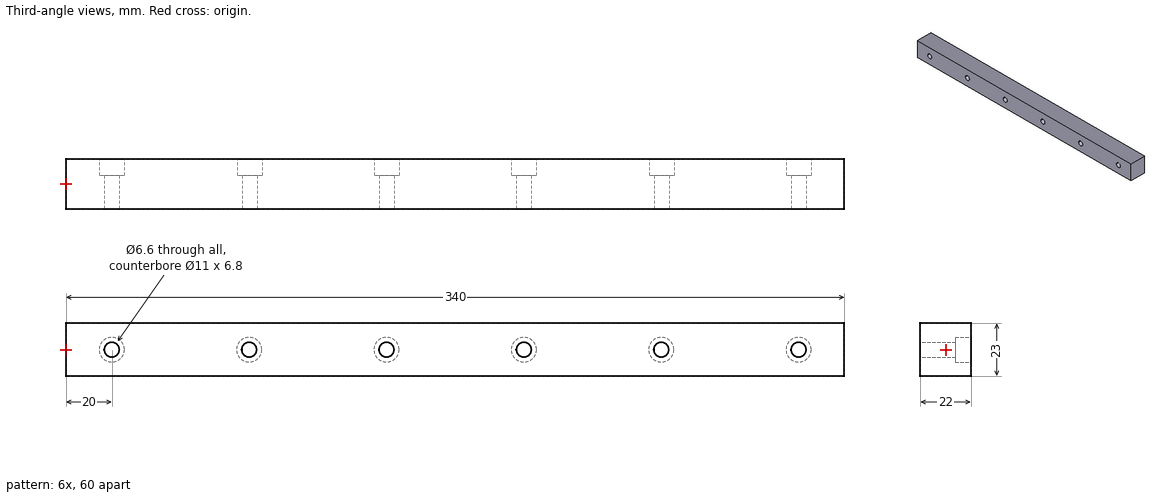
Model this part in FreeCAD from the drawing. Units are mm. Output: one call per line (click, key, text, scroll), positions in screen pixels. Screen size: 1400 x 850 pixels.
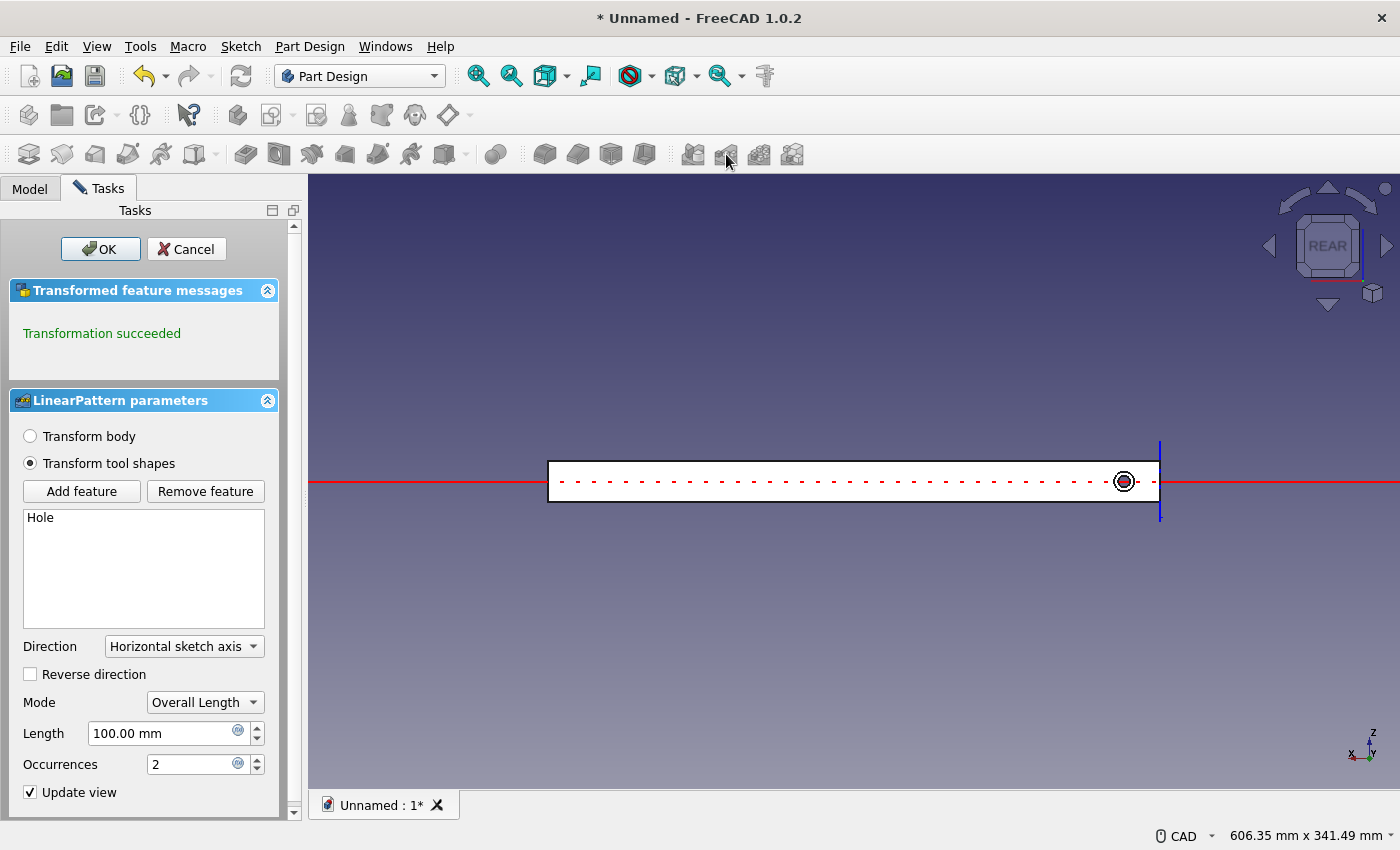
click(185, 646)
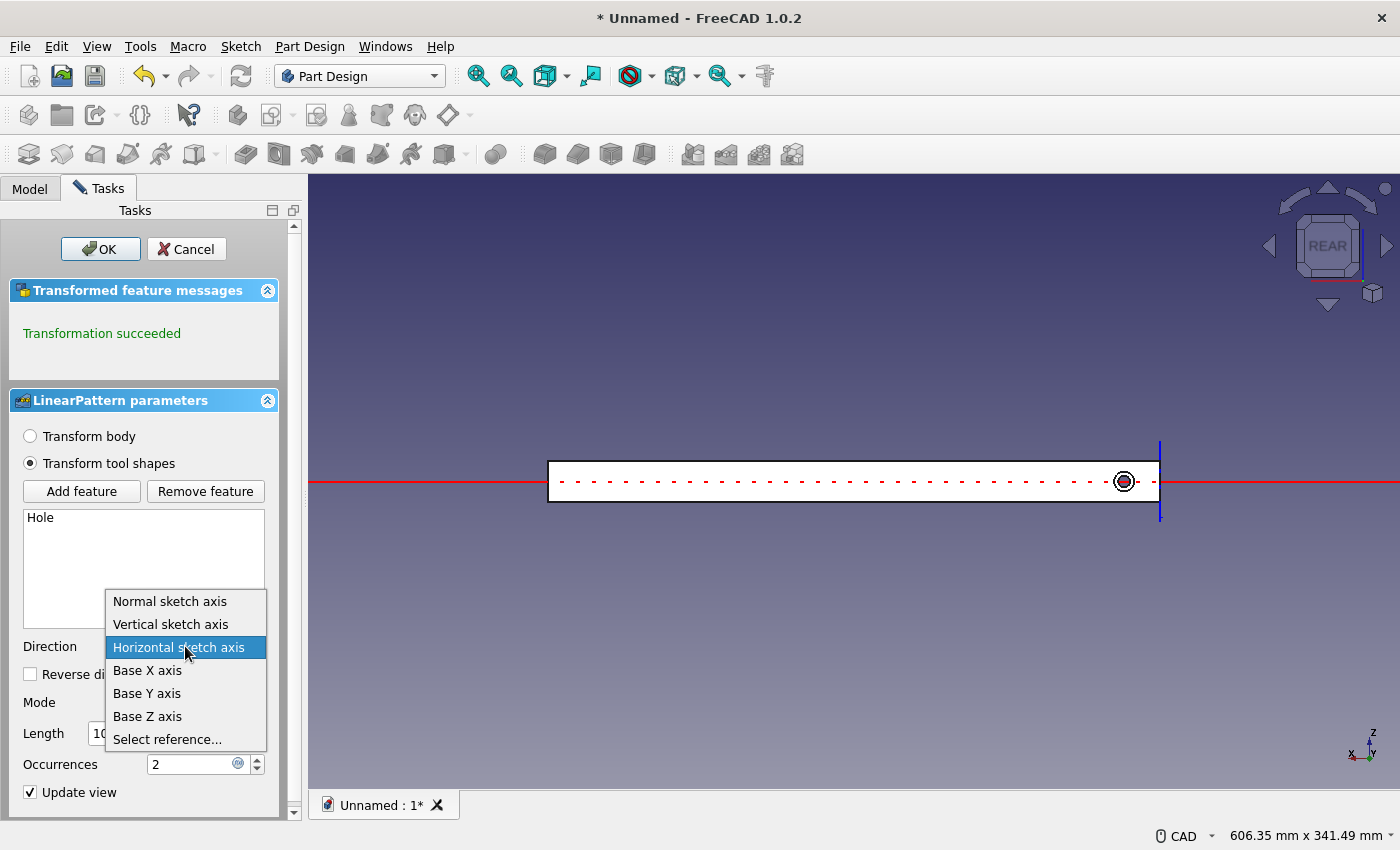
click(184, 670)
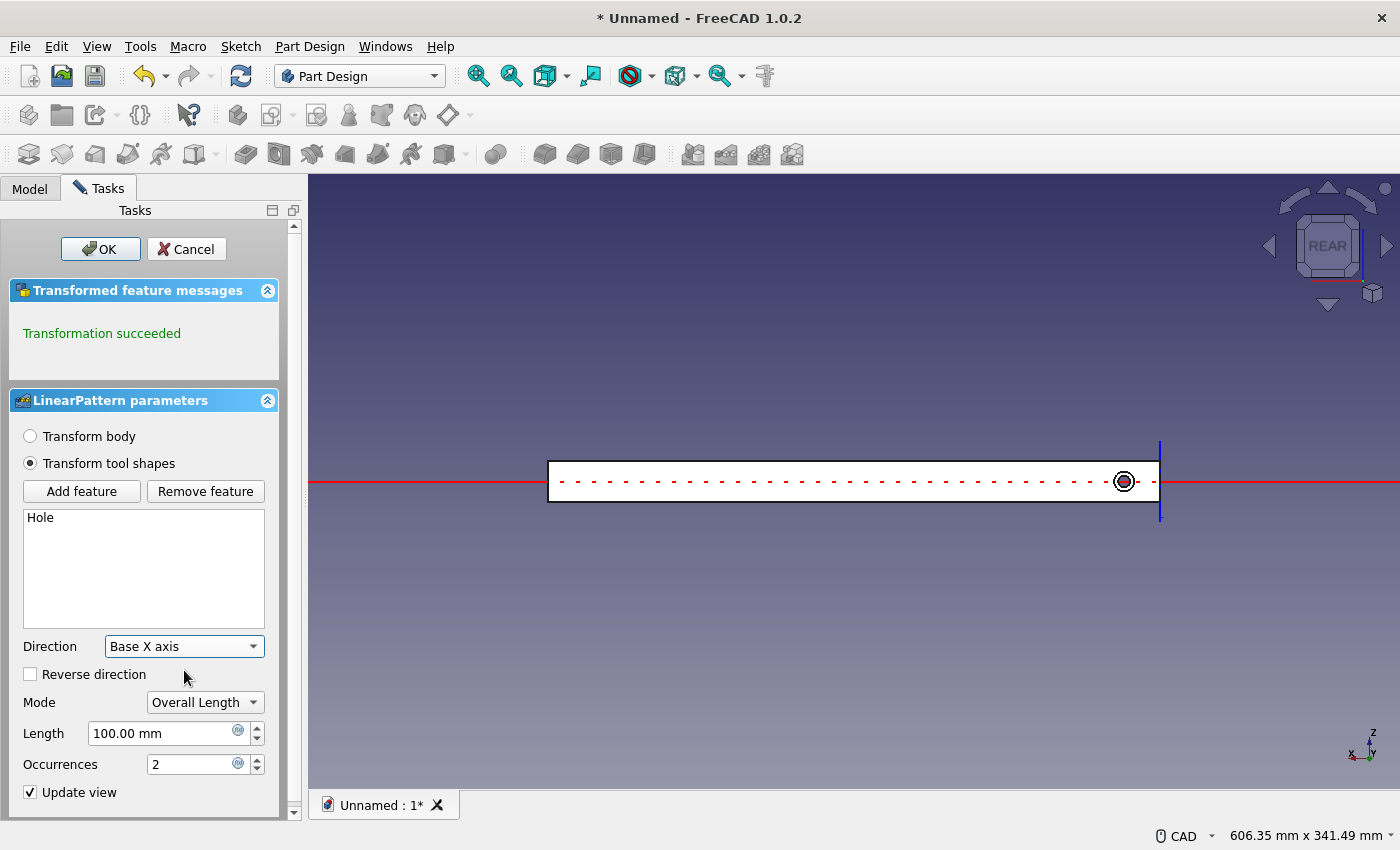
click(206, 702)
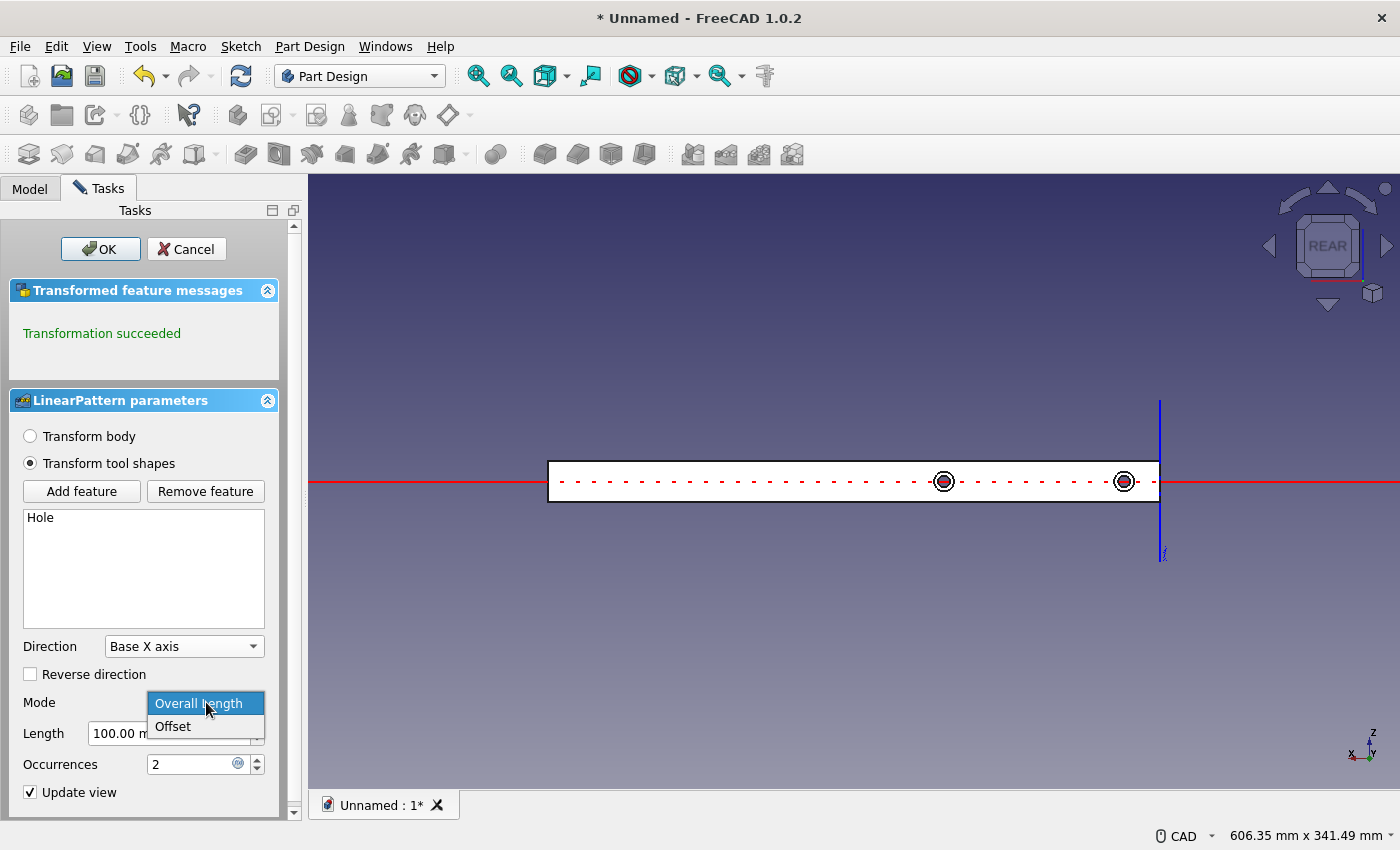
click(204, 726)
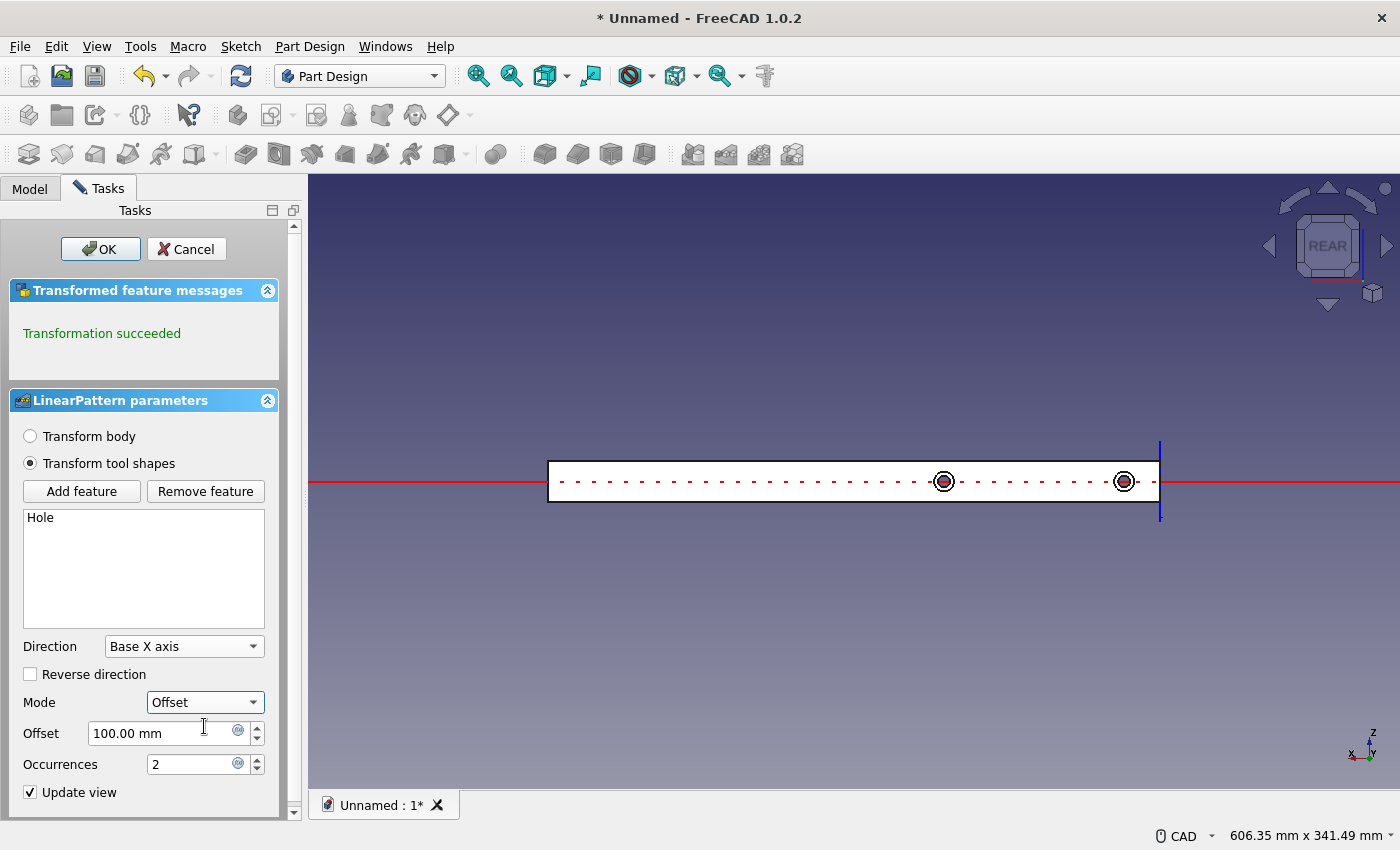
triple_click(170, 734)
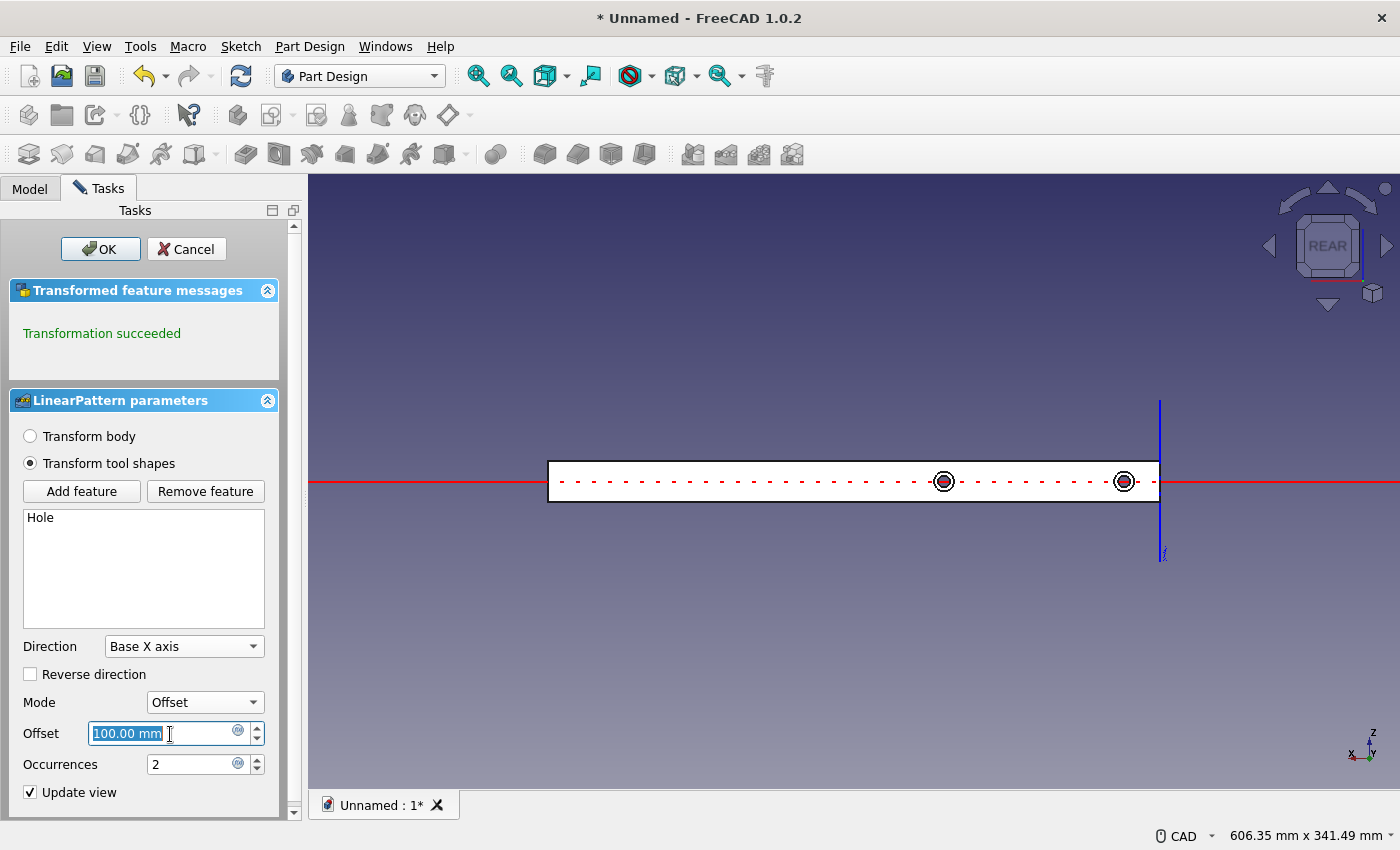
text(60)
key(Tab)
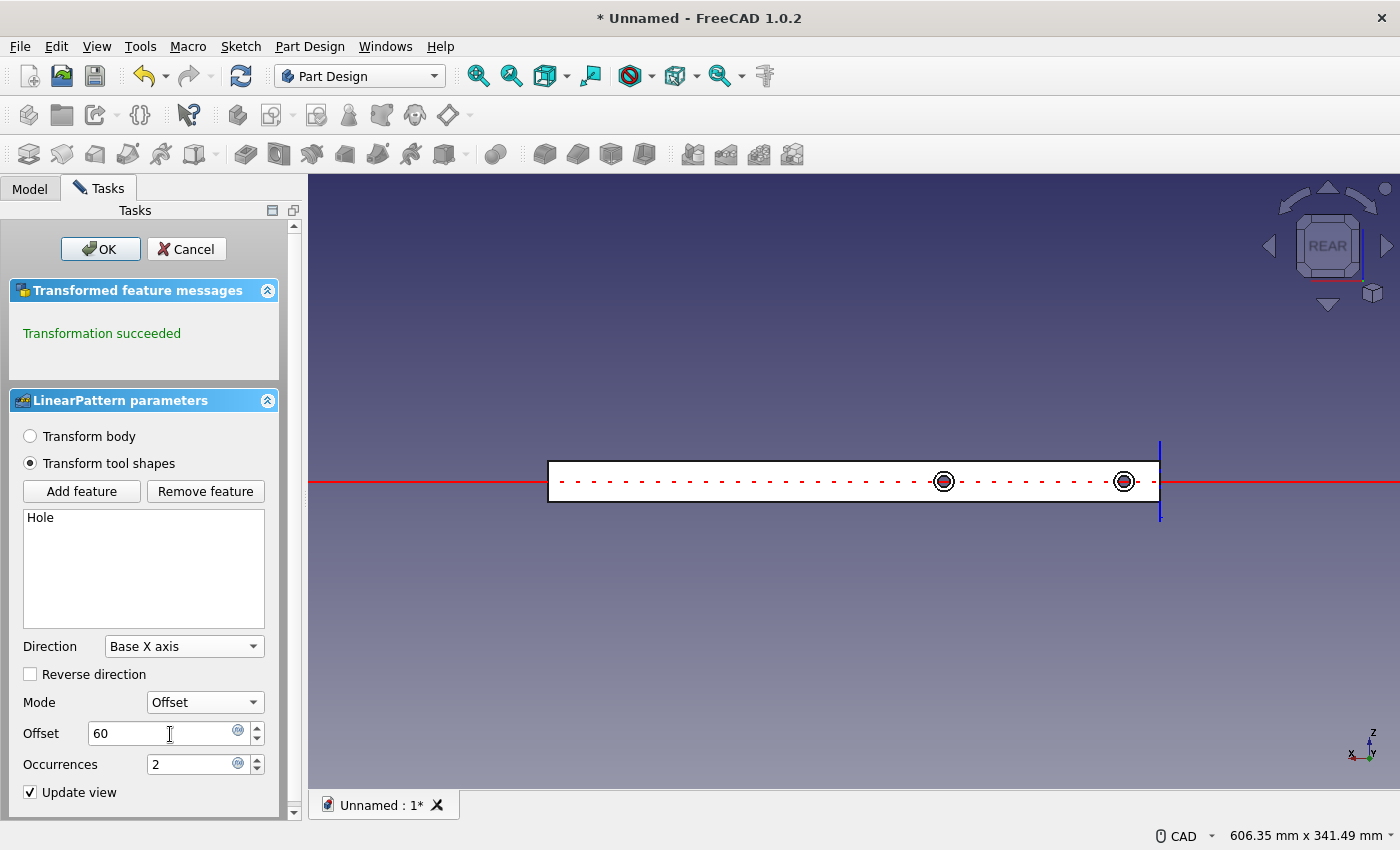
triple_click(199, 764)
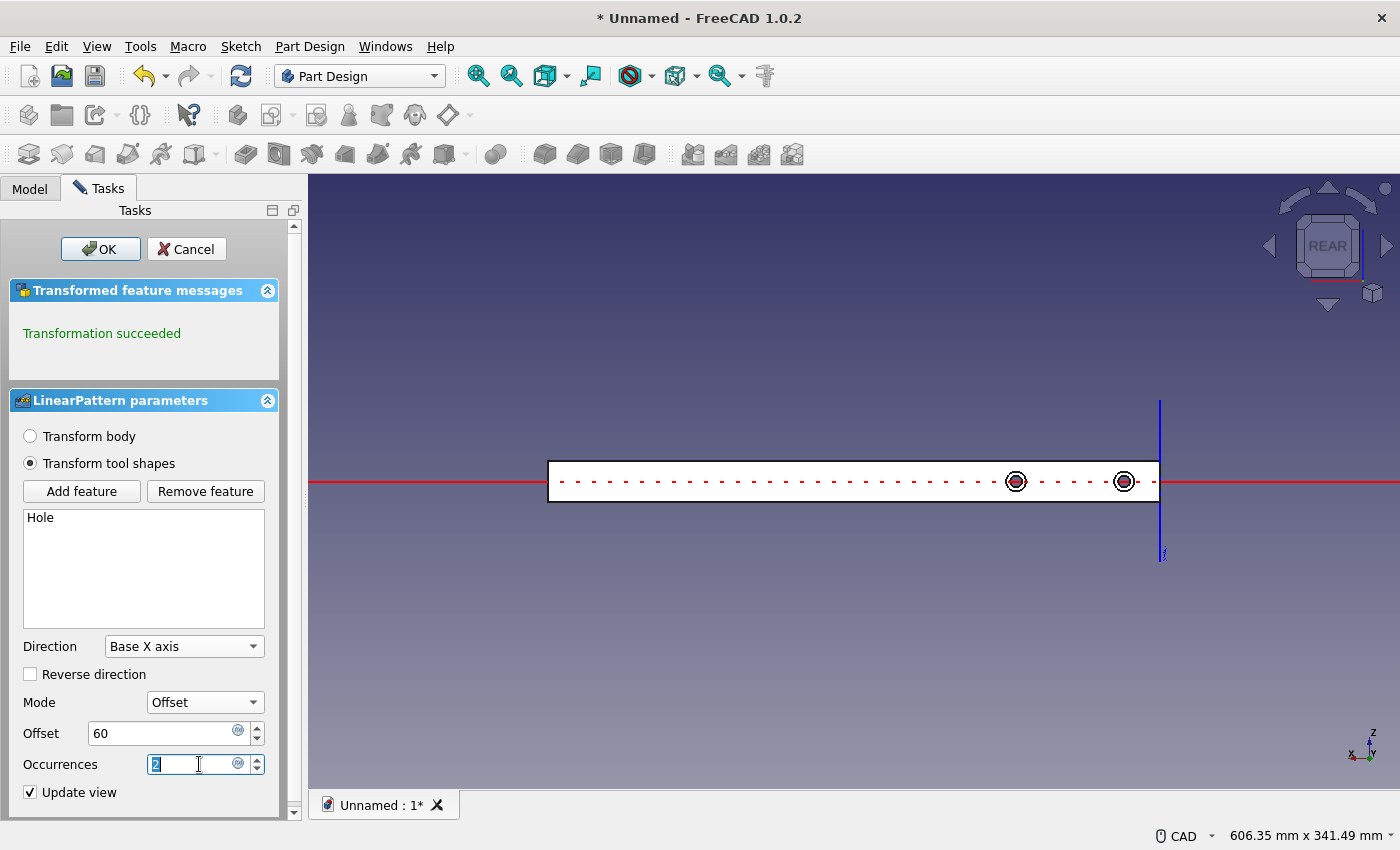
text(6)
key(Tab)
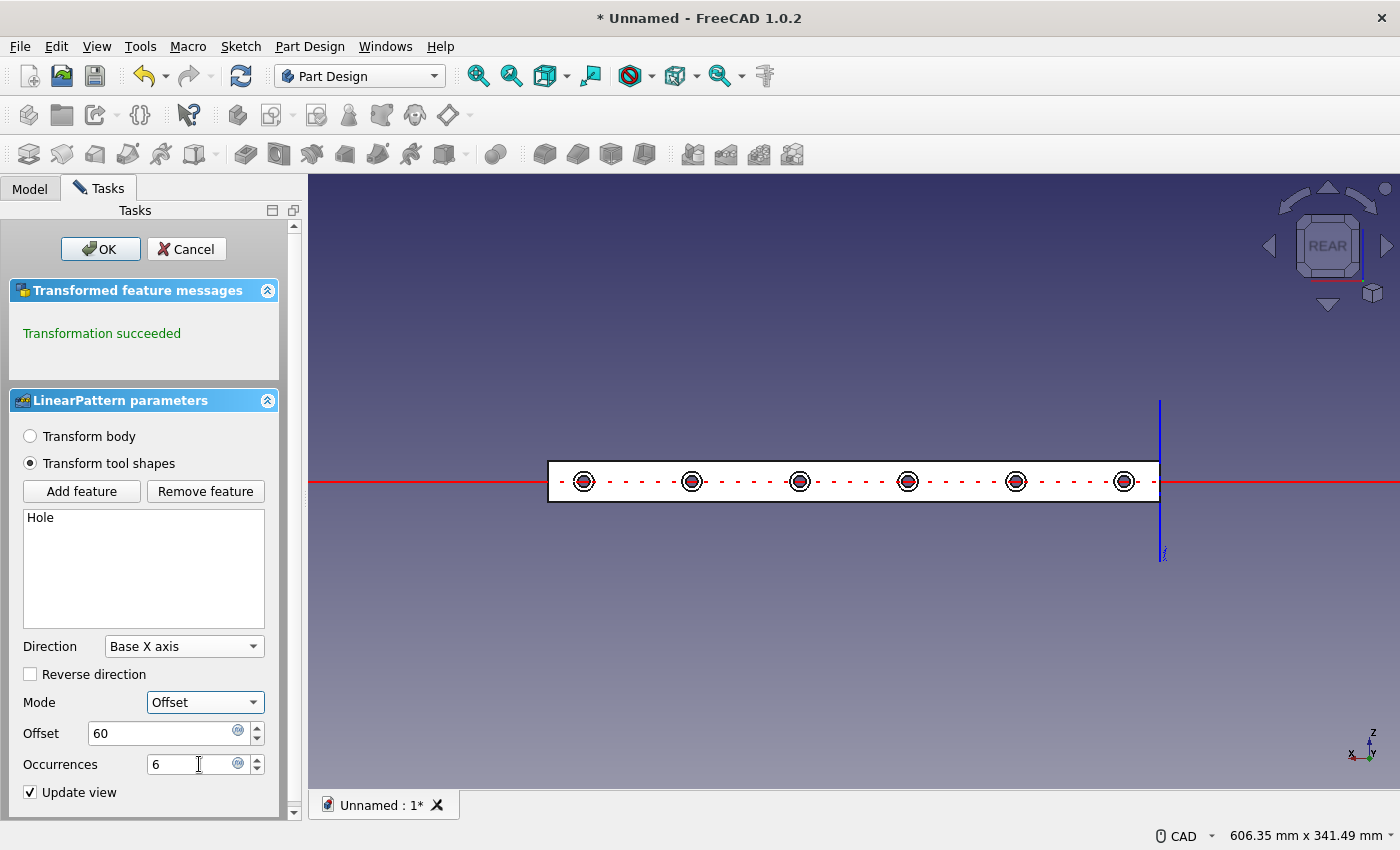
click(101, 249)